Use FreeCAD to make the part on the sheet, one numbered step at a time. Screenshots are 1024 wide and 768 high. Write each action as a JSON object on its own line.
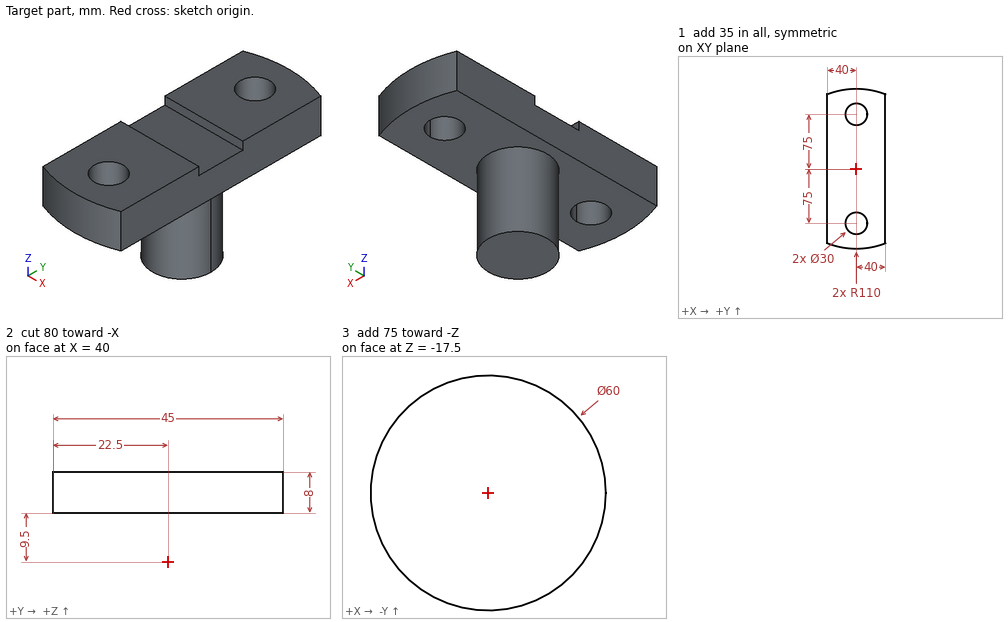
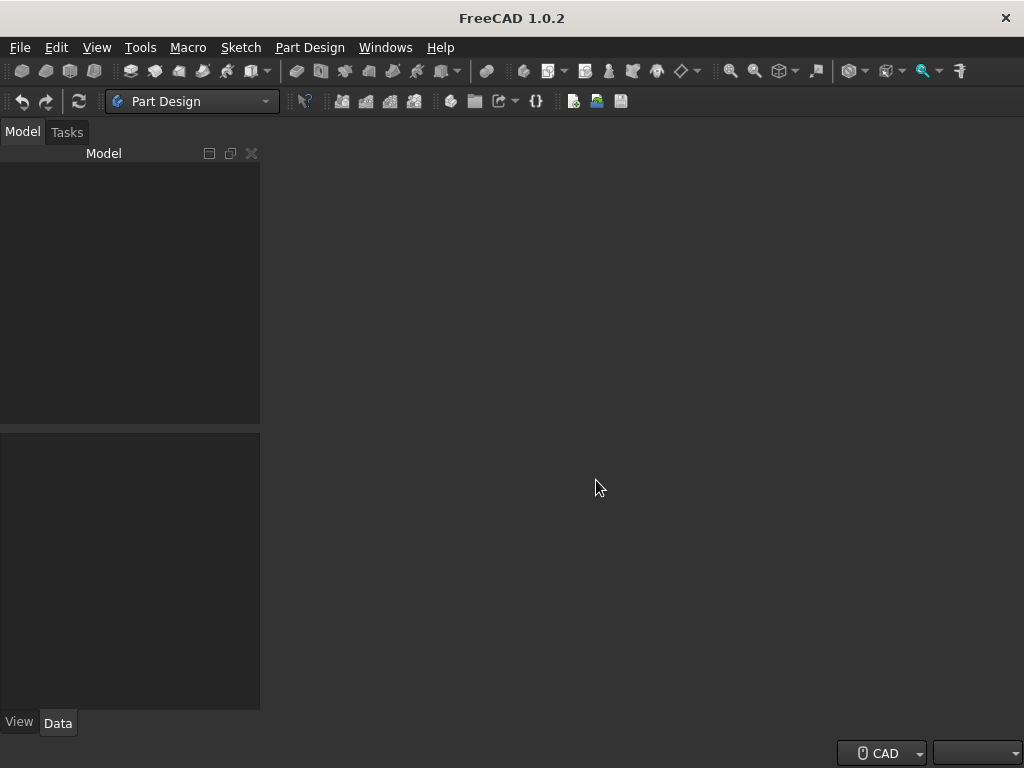
{"action": "key", "text": "ctrl+n"}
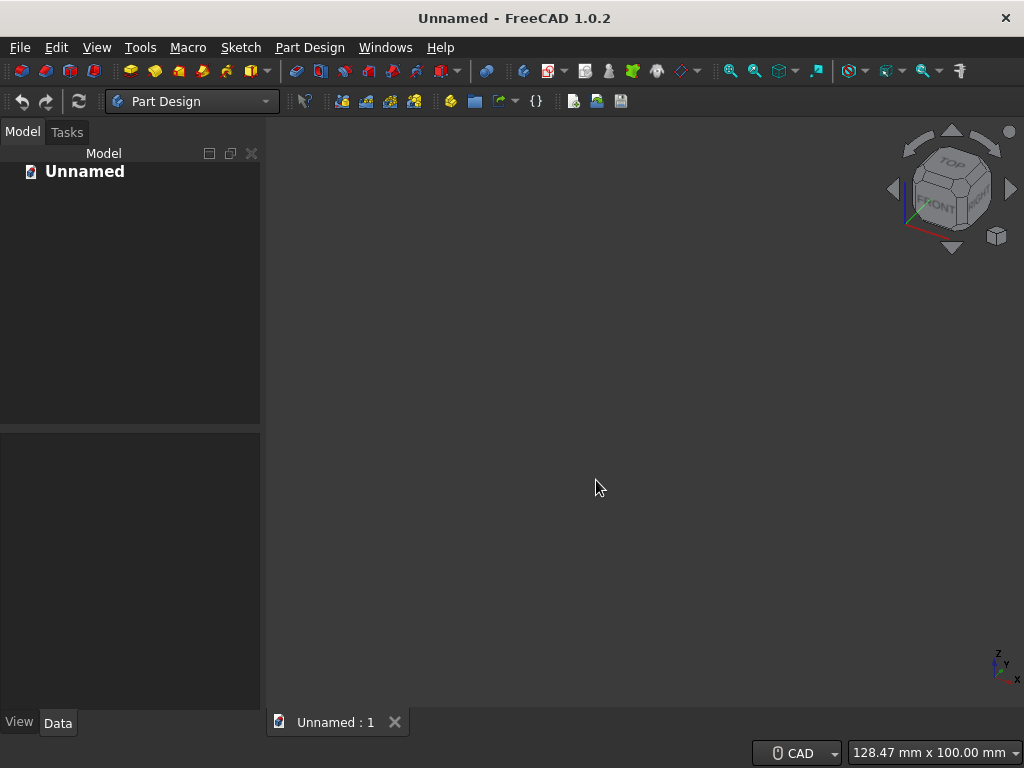
{"action": "left_click", "coordinate": [548, 72]}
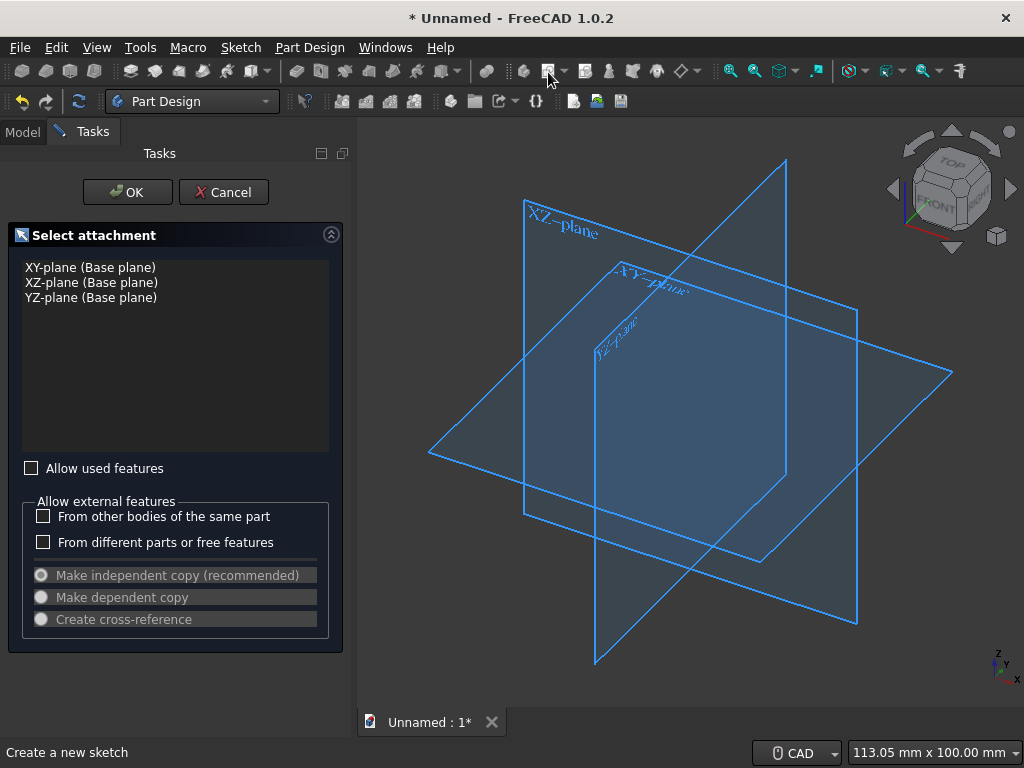
{"action": "left_click", "coordinate": [82, 268]}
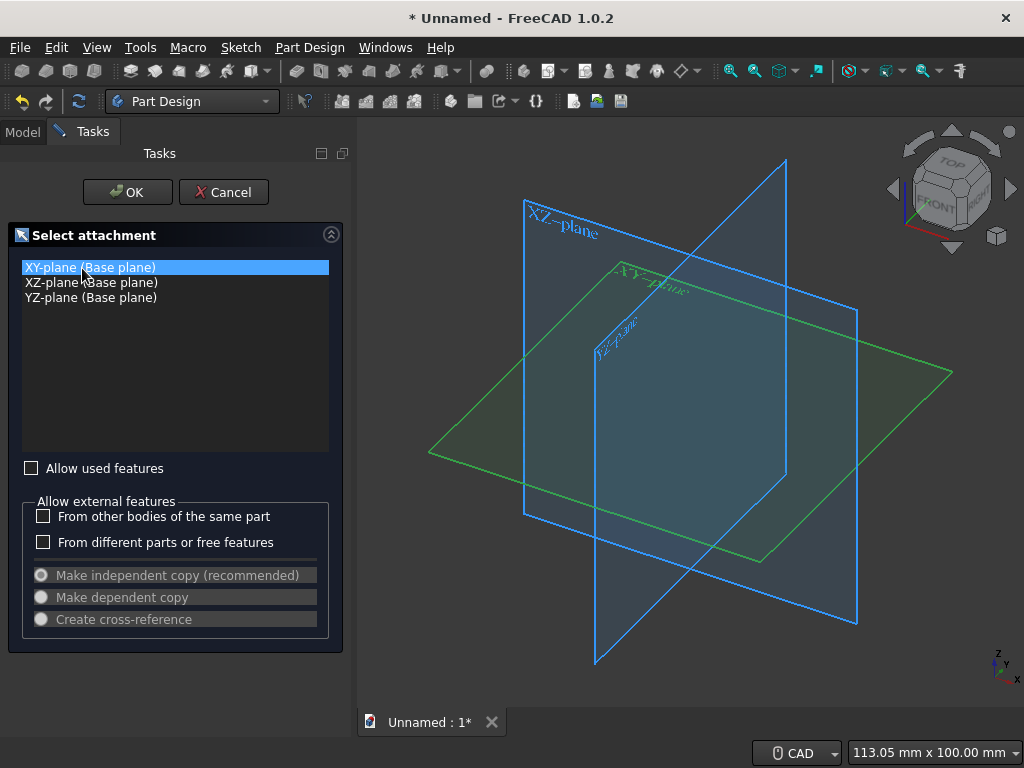
{"action": "left_click", "coordinate": [128, 192]}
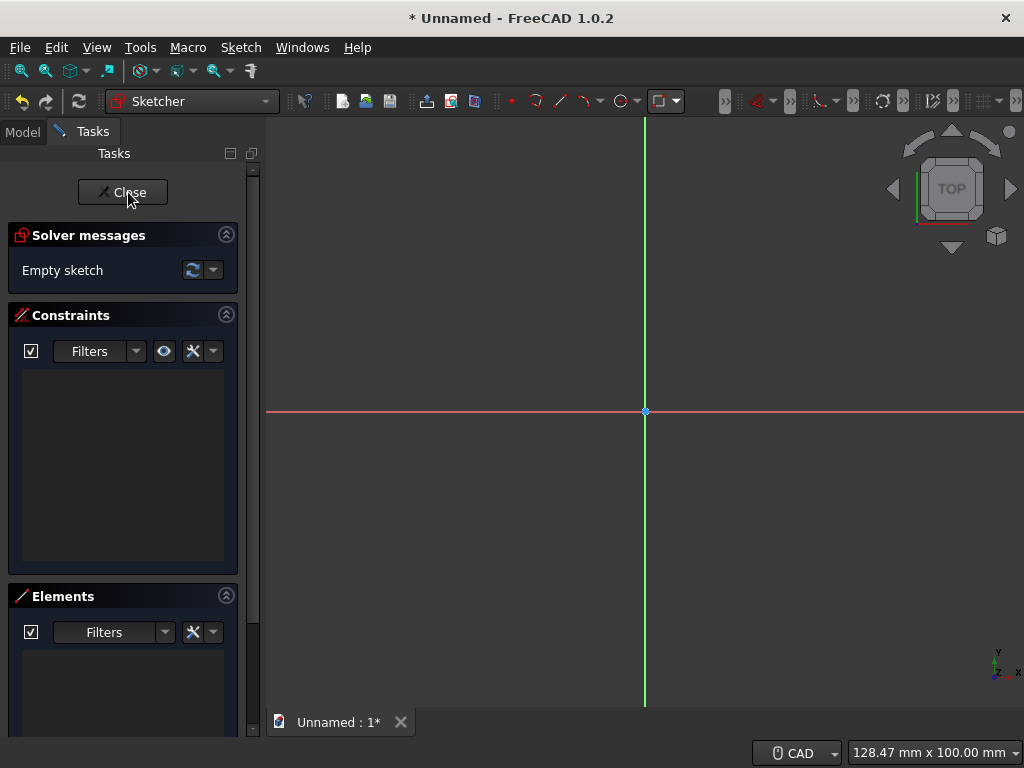
{"action": "scroll", "coordinate": [547, 412], "scroll_direction": "down", "scroll_amount": 6}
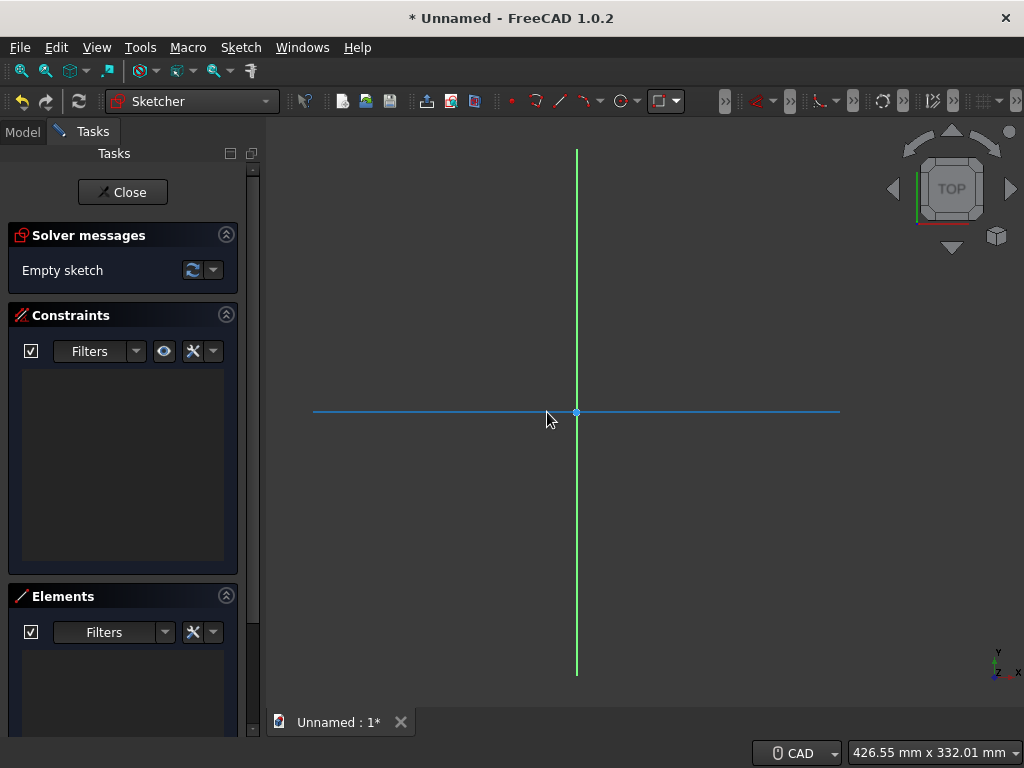
{"action": "left_click", "coordinate": [560, 102]}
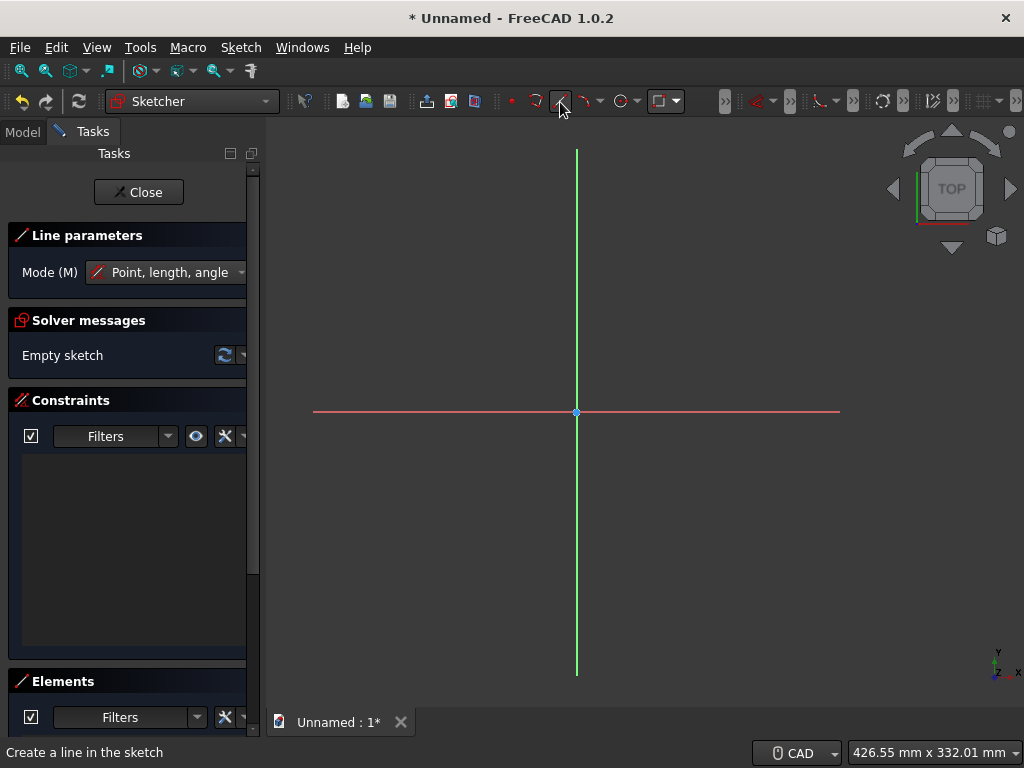
{"action": "left_click", "coordinate": [506, 230]}
{"action": "left_click", "coordinate": [506, 594]}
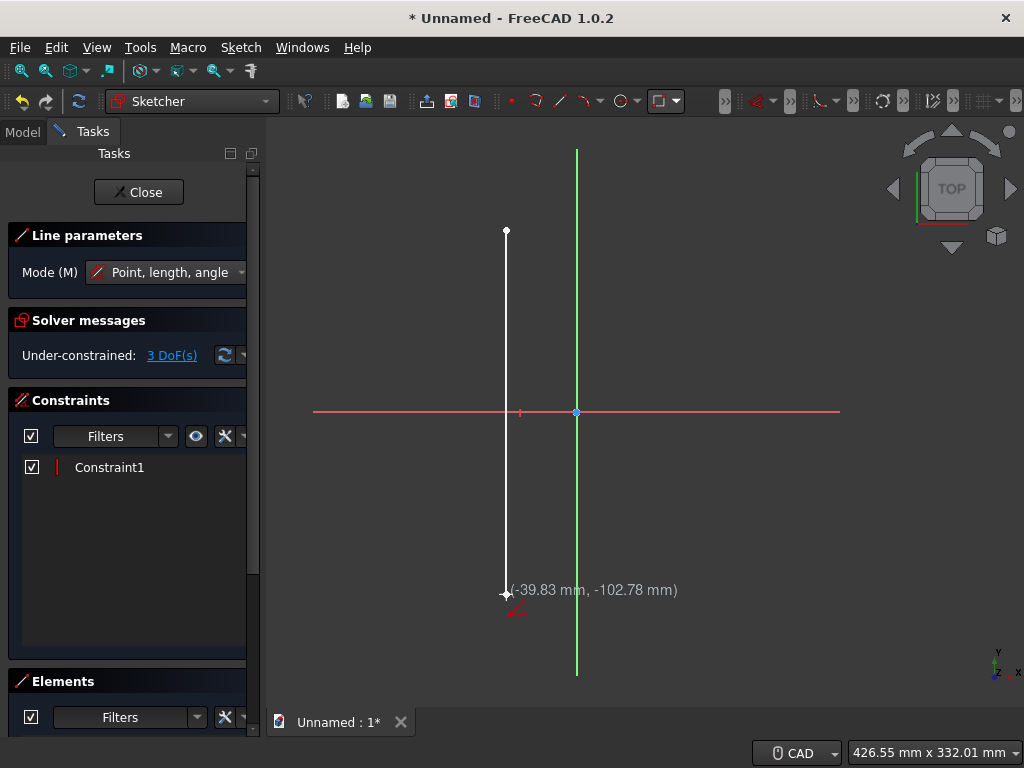
{"action": "left_click", "coordinate": [648, 594]}
{"action": "left_click", "coordinate": [648, 230]}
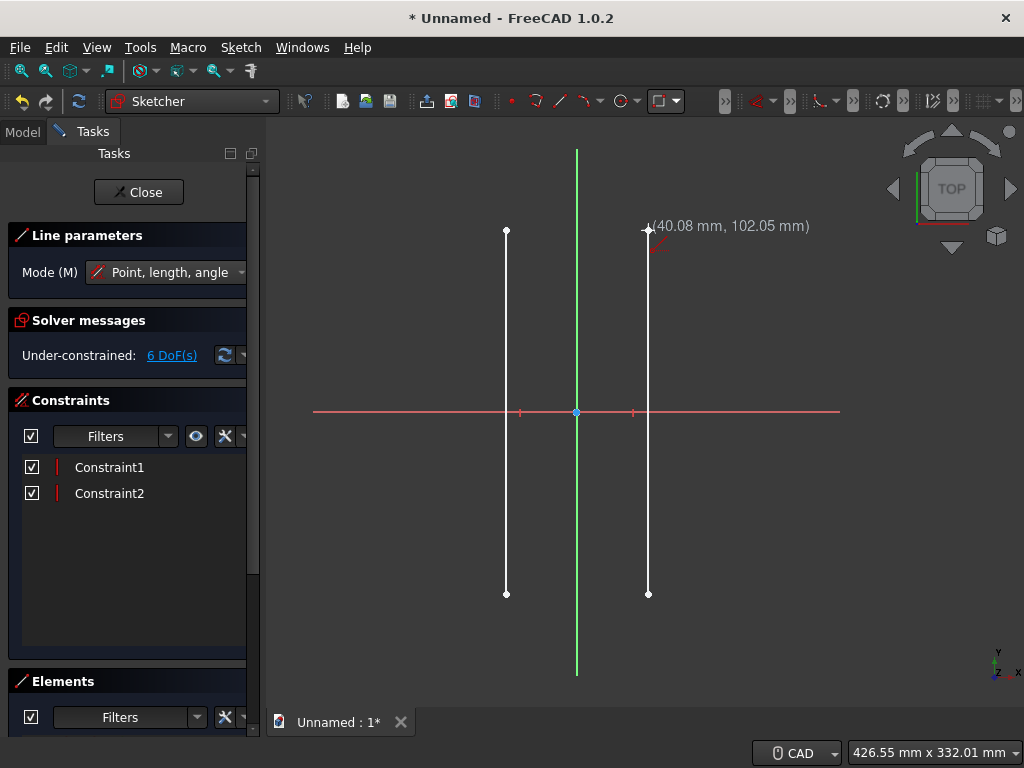
{"action": "left_click", "coordinate": [584, 102]}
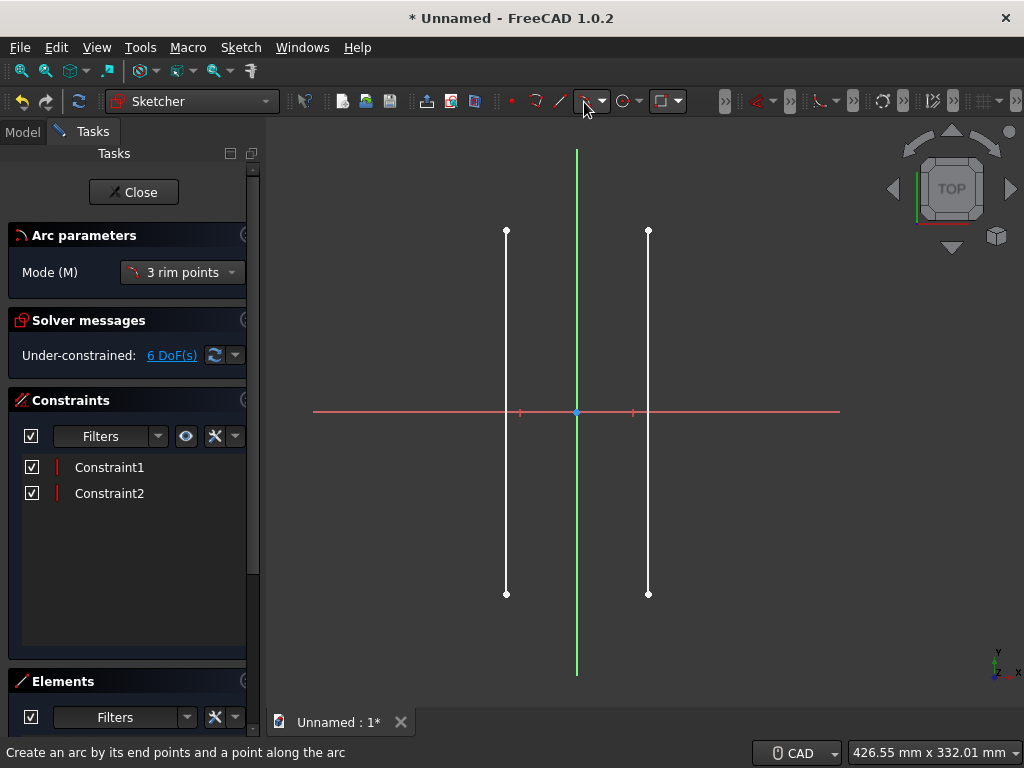
{"action": "left_click", "coordinate": [506, 595]}
{"action": "left_click", "coordinate": [648, 595]}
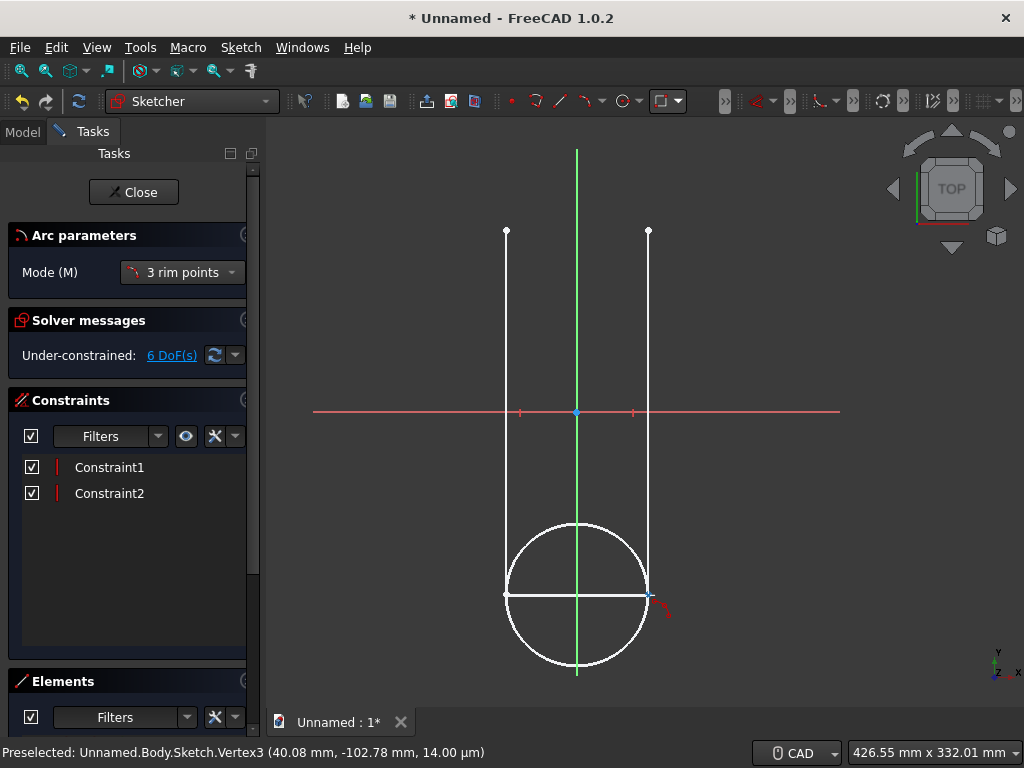
{"action": "scroll", "coordinate": [562, 607], "scroll_direction": "up", "scroll_amount": 2}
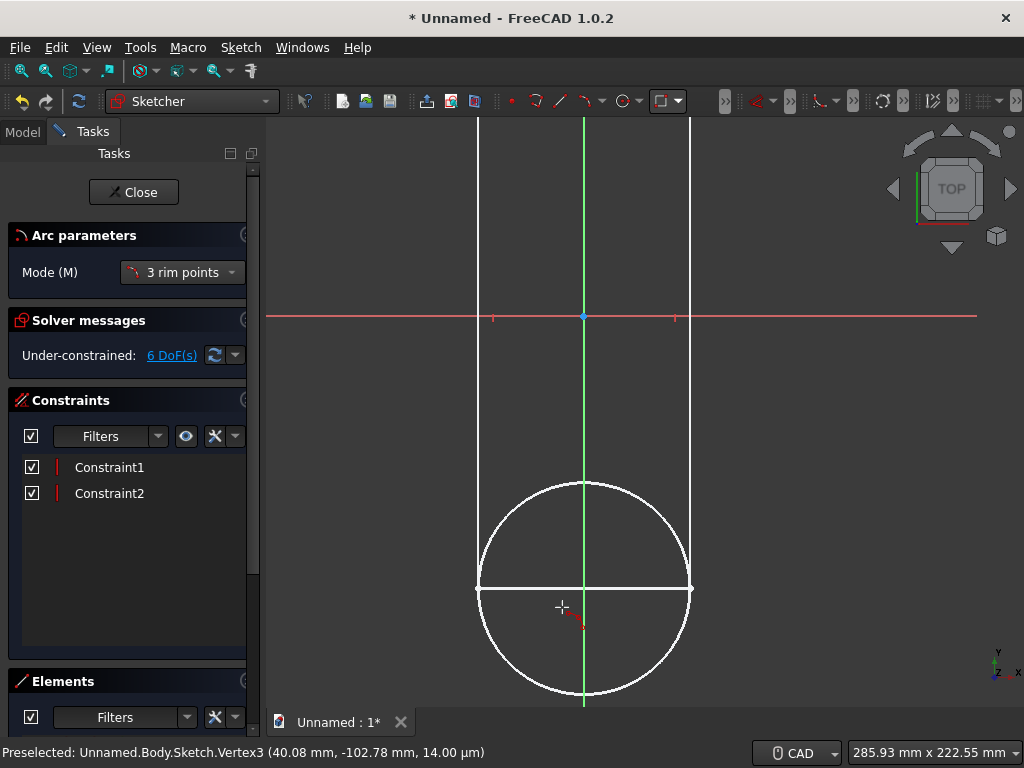
{"action": "left_click", "coordinate": [562, 607]}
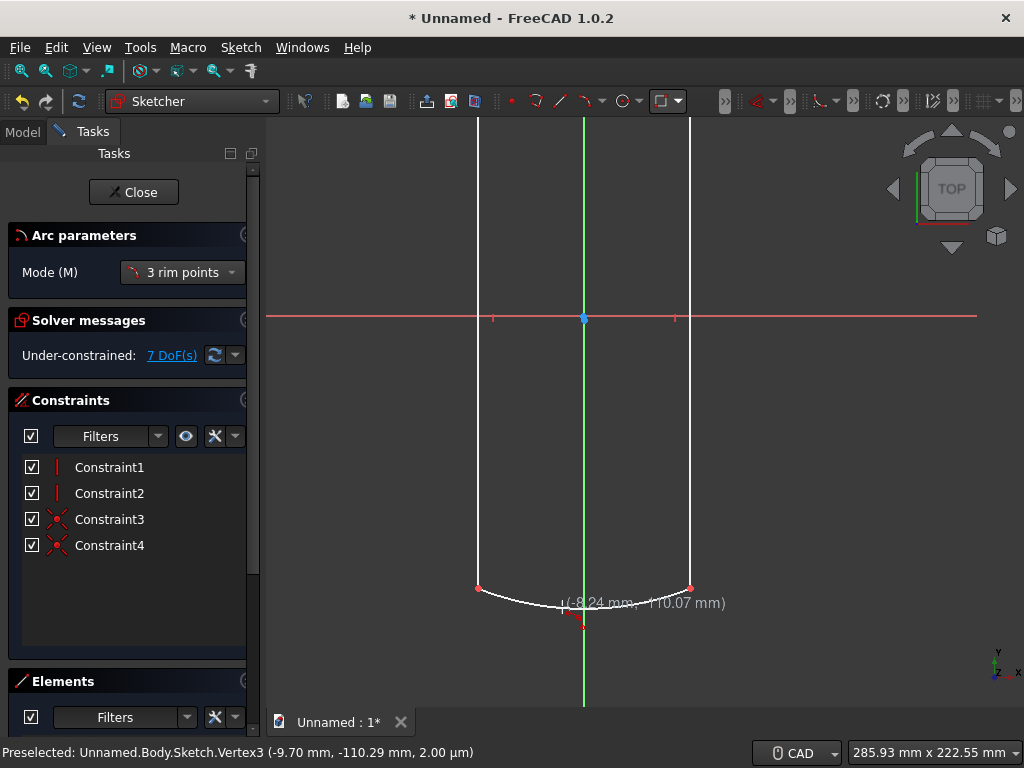
{"action": "scroll", "coordinate": [562, 607], "scroll_direction": "down", "scroll_amount": 2}